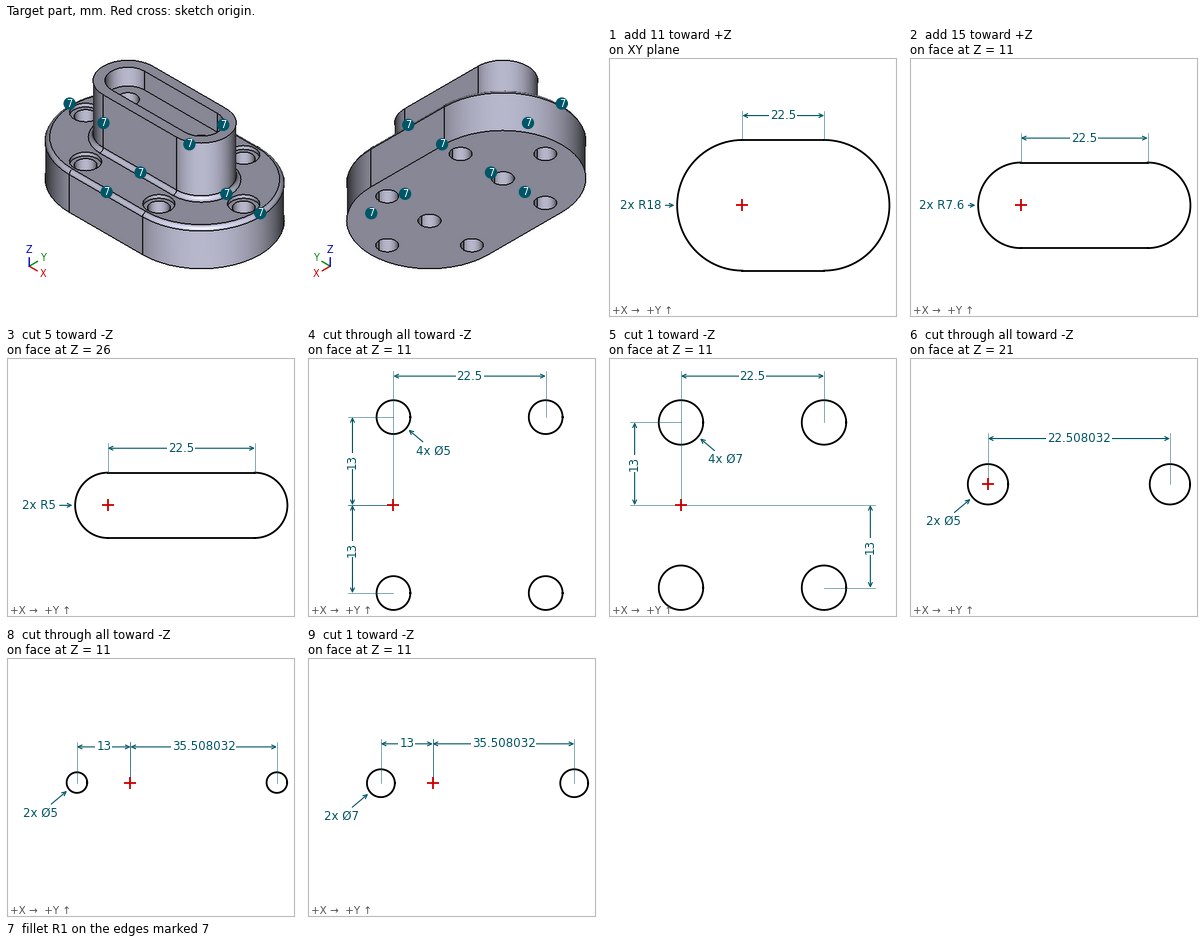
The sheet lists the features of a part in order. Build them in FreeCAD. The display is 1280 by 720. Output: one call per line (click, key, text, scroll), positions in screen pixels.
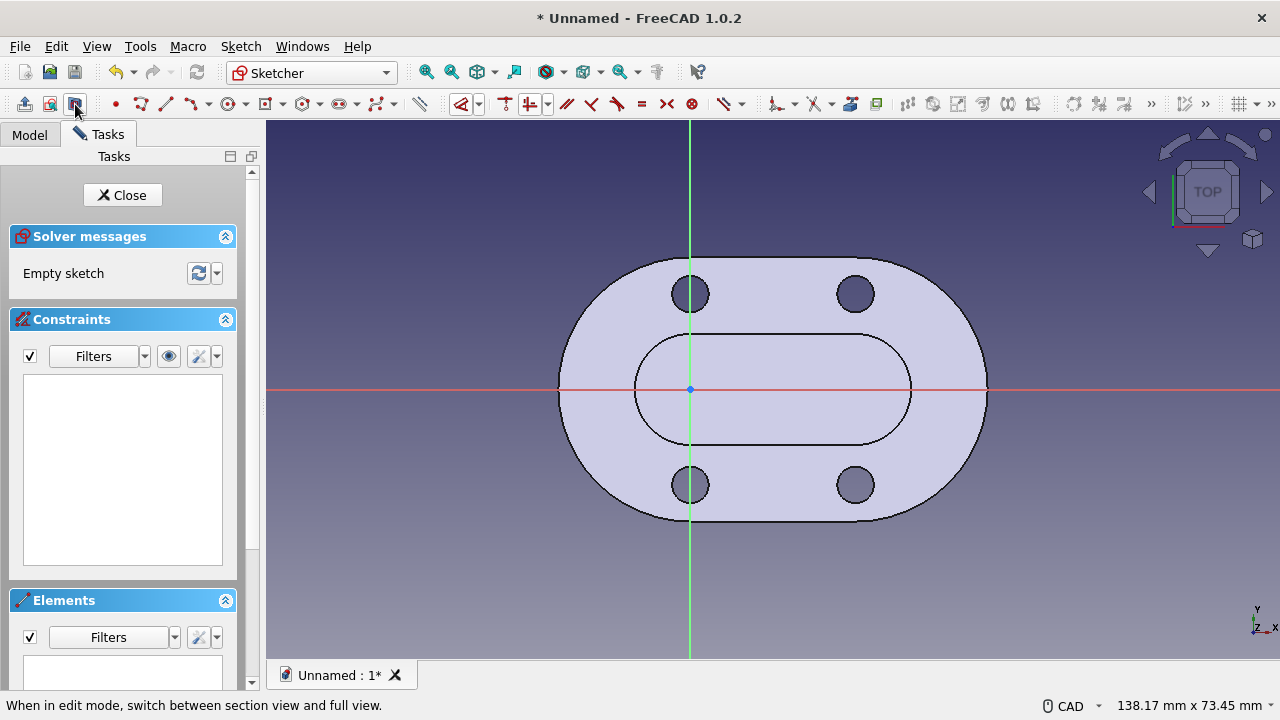
scroll(912, 390, up, 2)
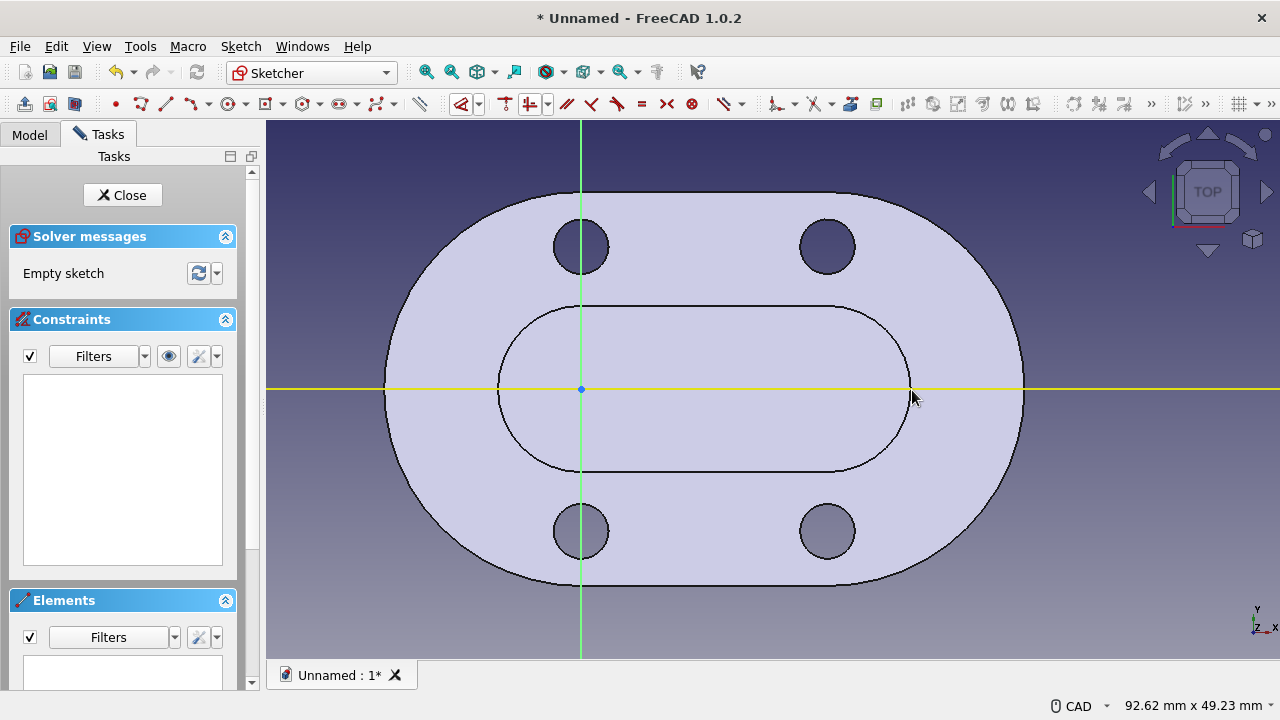
key(g)
key(c)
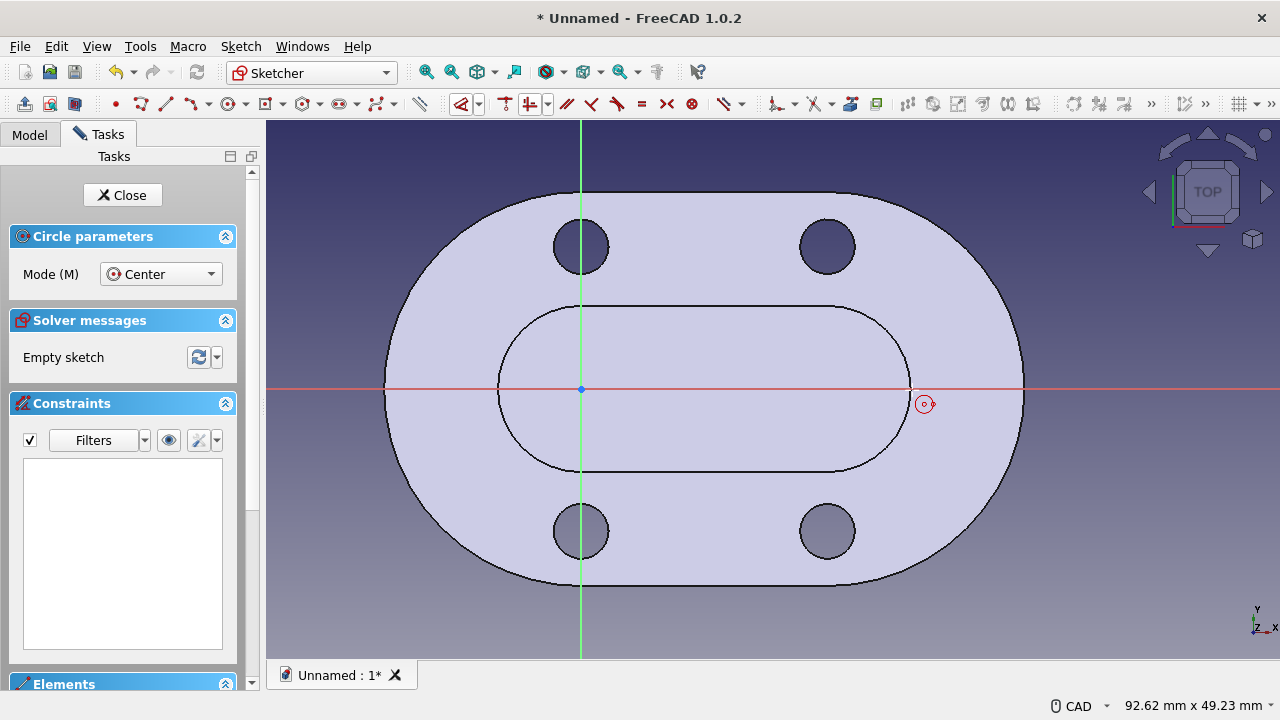
click(581, 247)
move(608, 220)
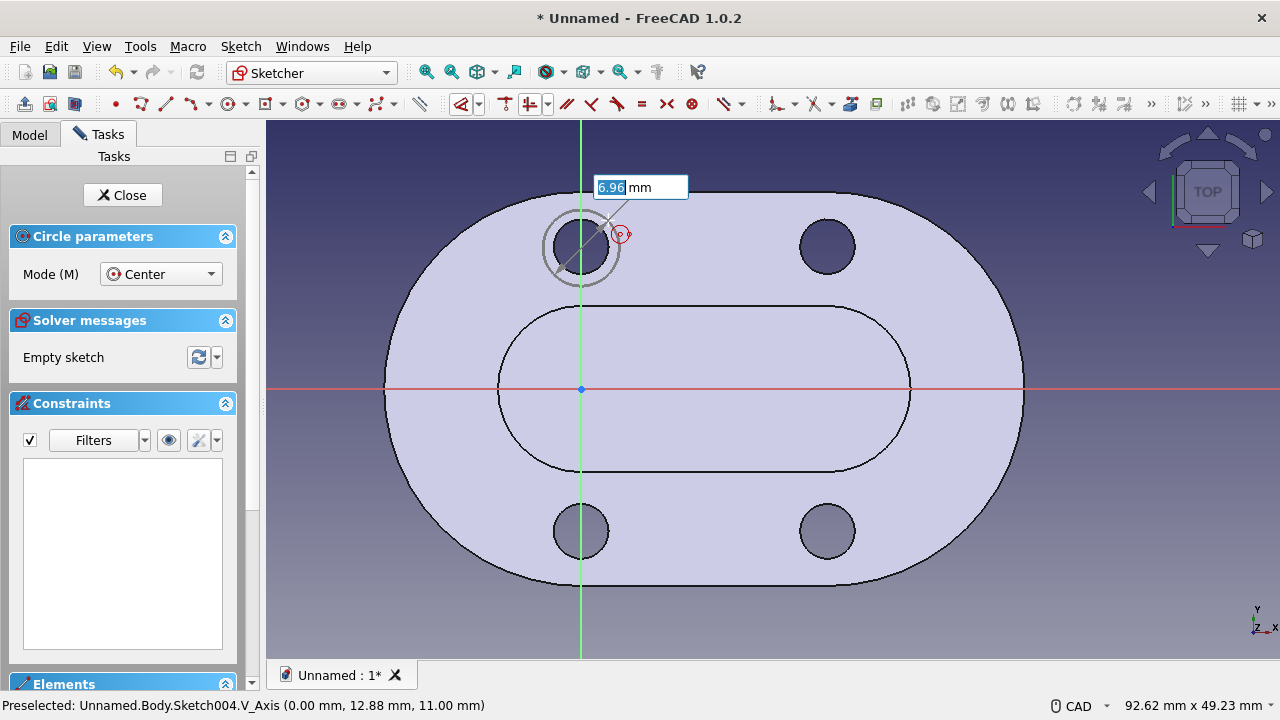
text(7)
key(Return)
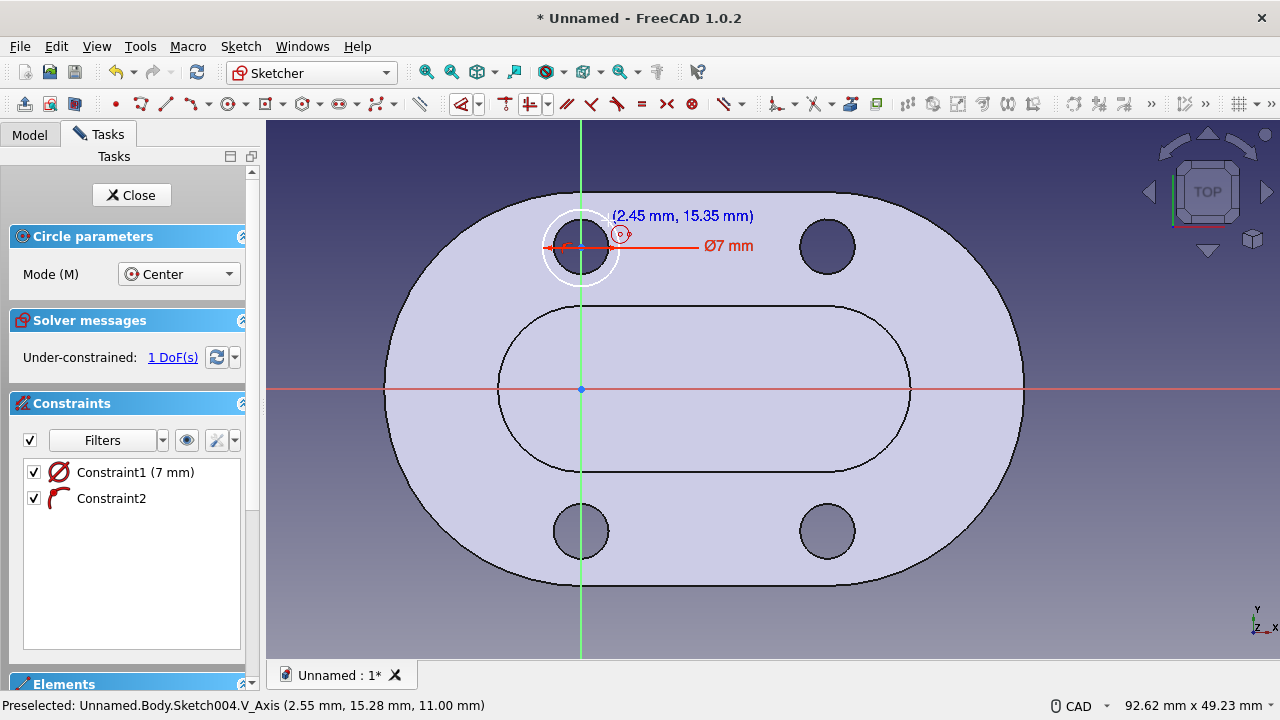
click(827, 247)
move(855, 220)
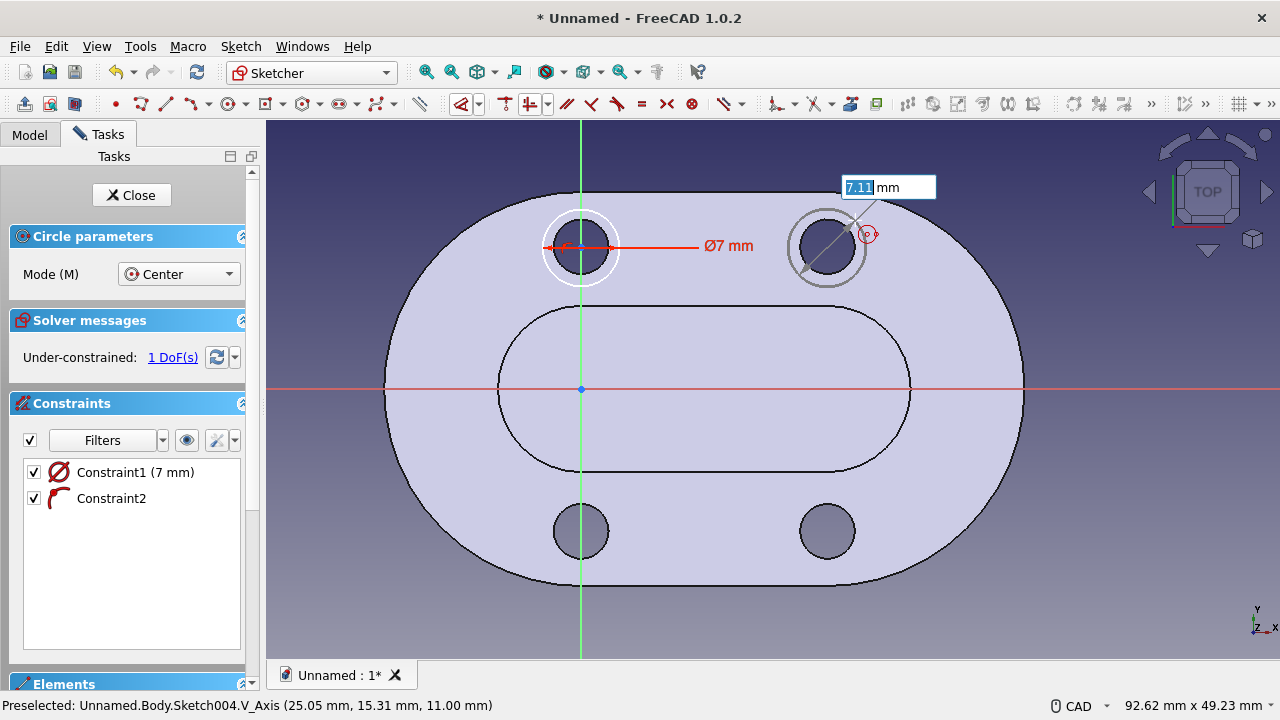
text(7)
key(Return)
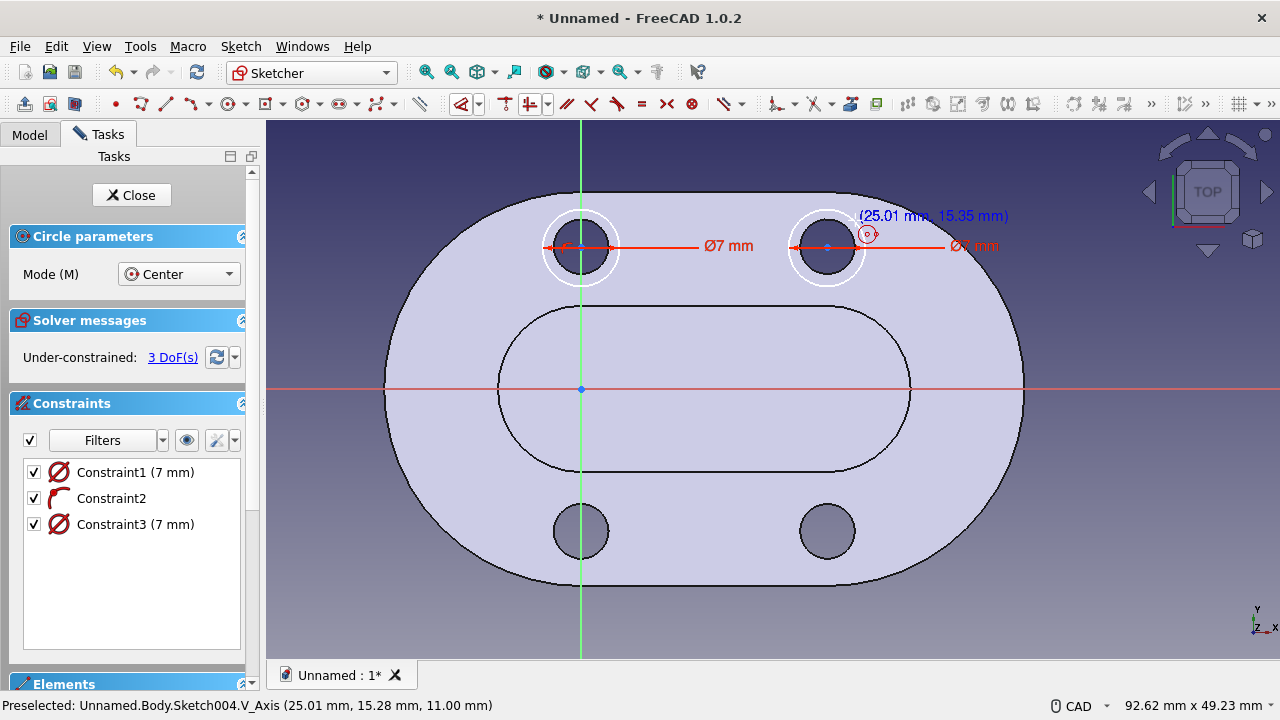
click(827, 531)
move(855, 504)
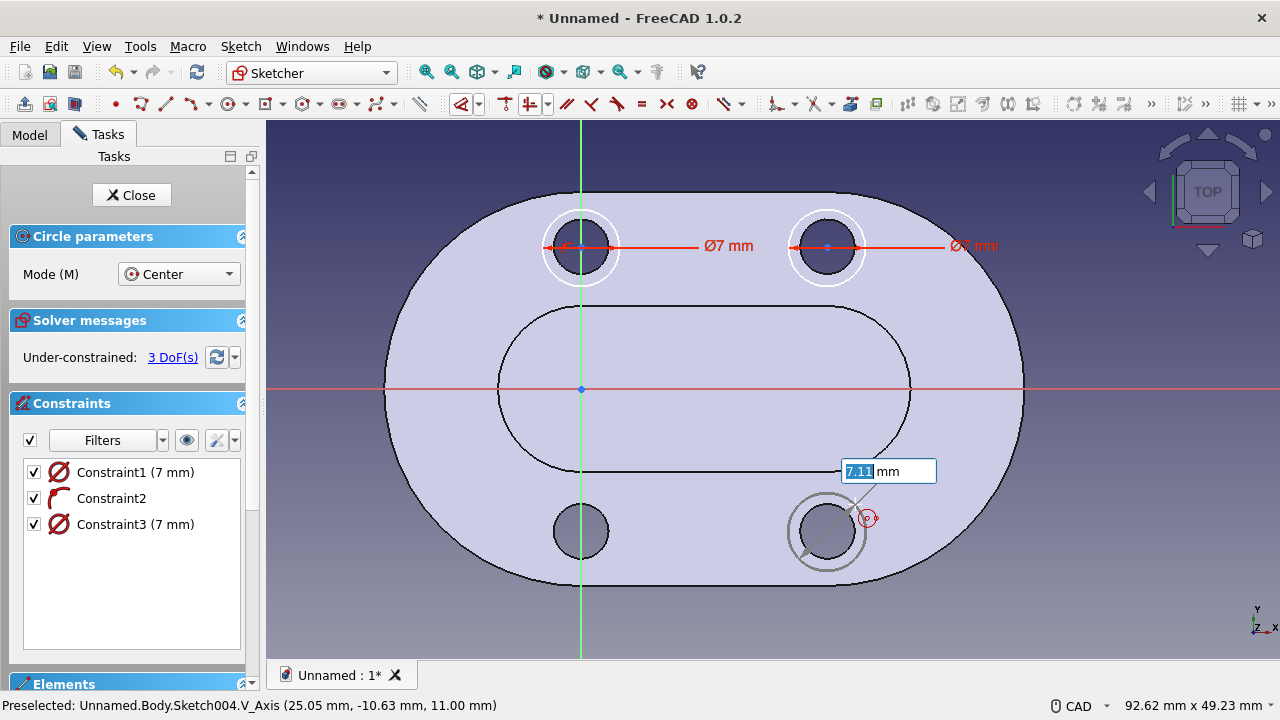
text(7)
key(Return)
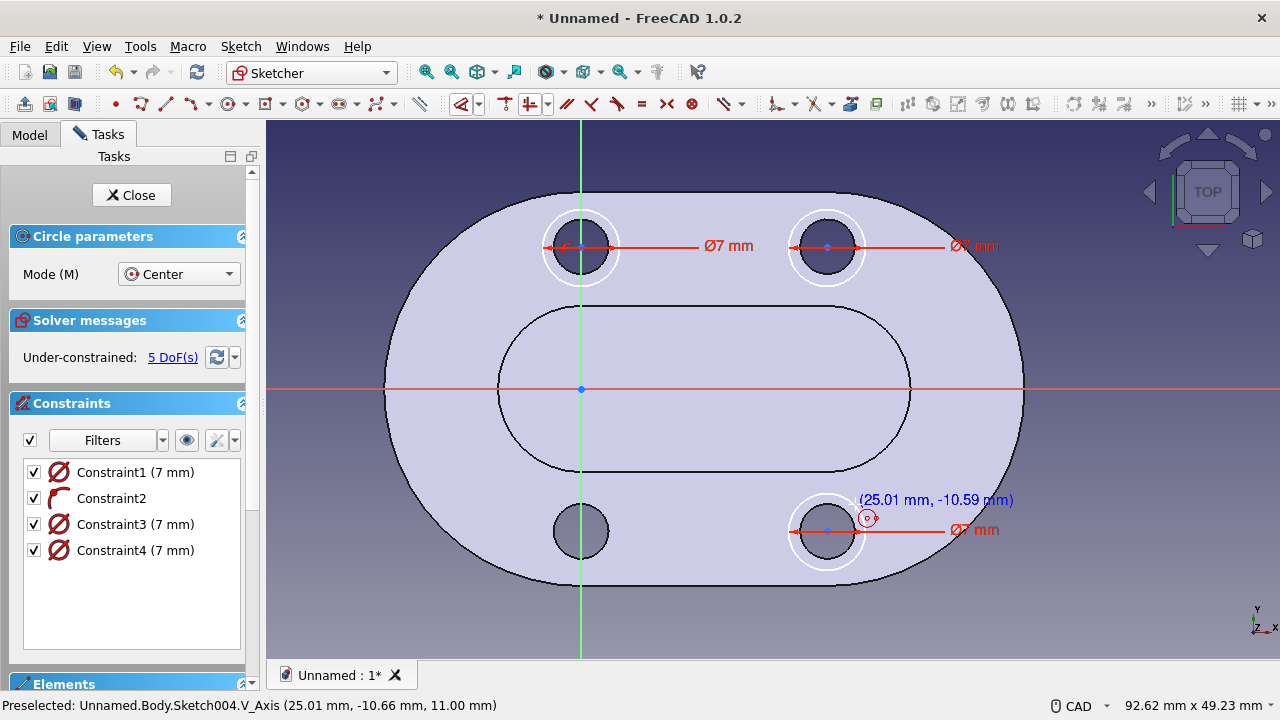
click(581, 531)
move(608, 504)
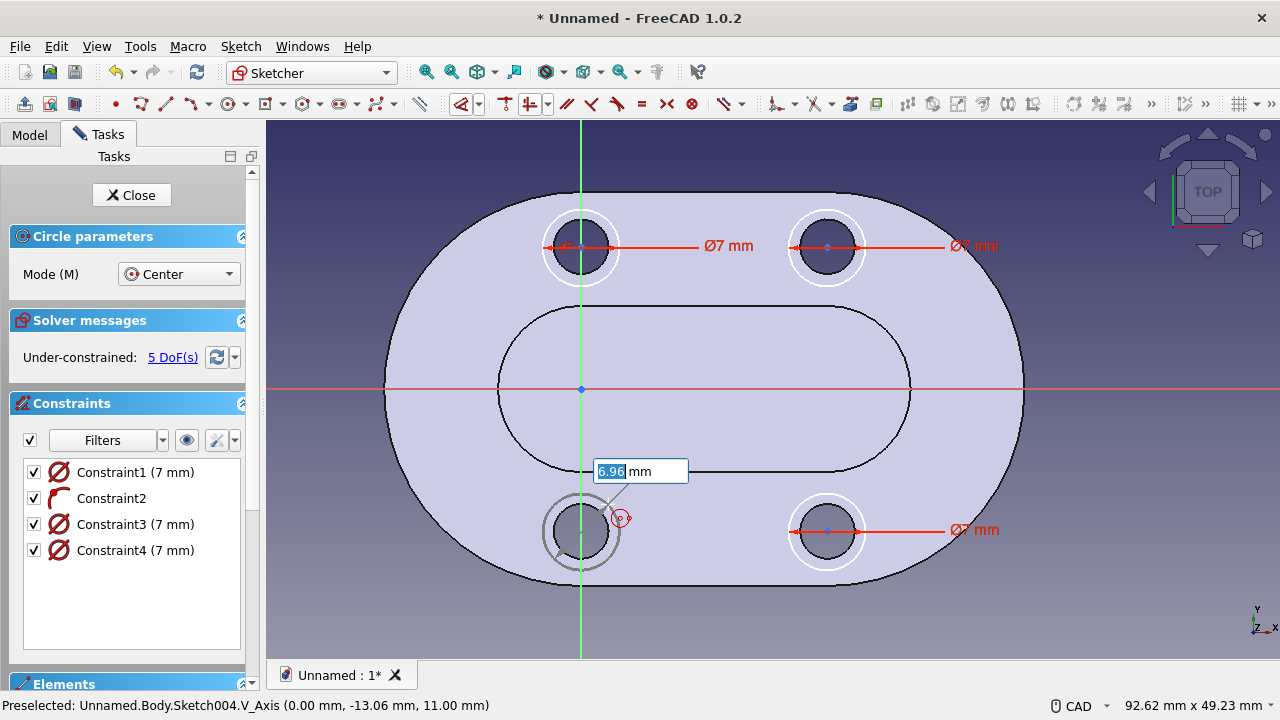
text(7)
key(Return)
key(Escape)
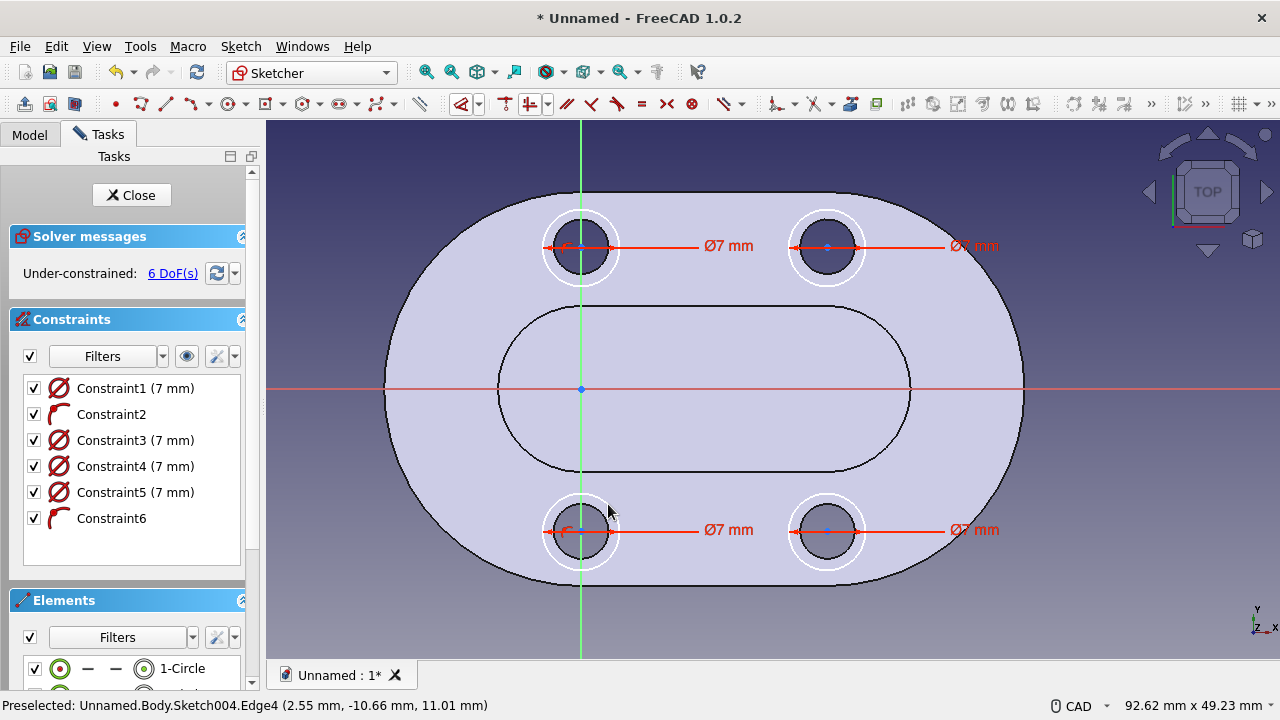
click(581, 248)